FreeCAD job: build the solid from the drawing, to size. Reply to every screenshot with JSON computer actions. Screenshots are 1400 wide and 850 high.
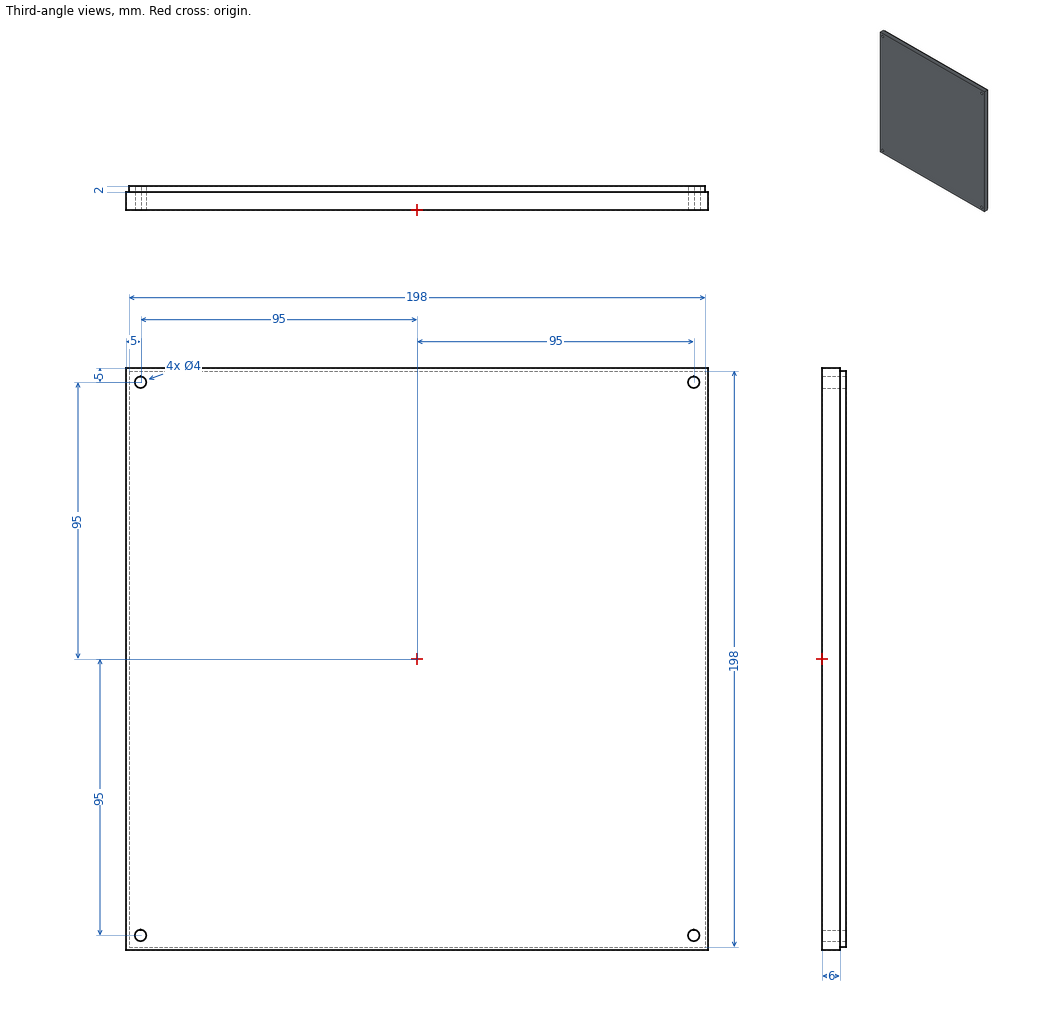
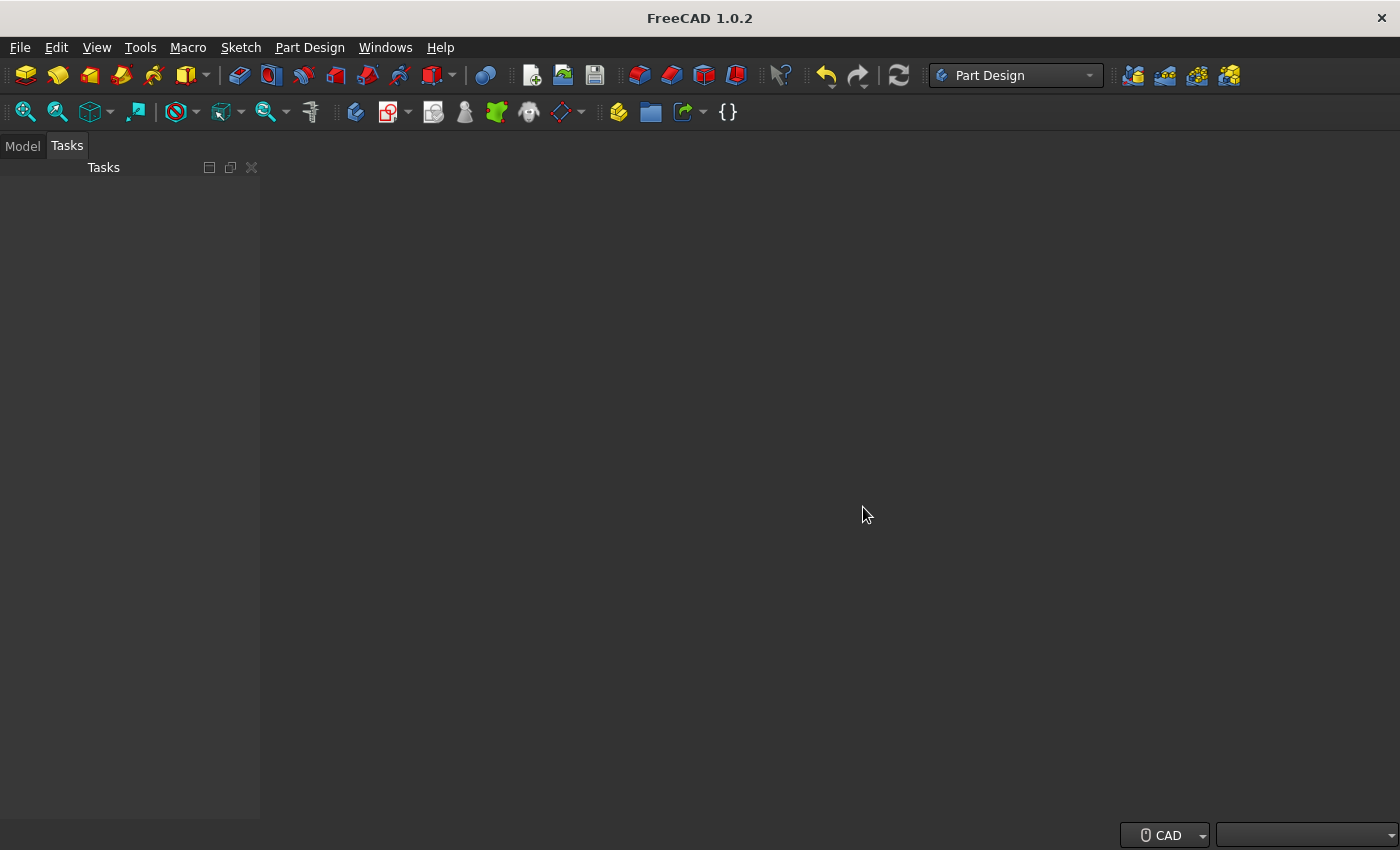
{"action": "left_click", "coordinate": [532, 76]}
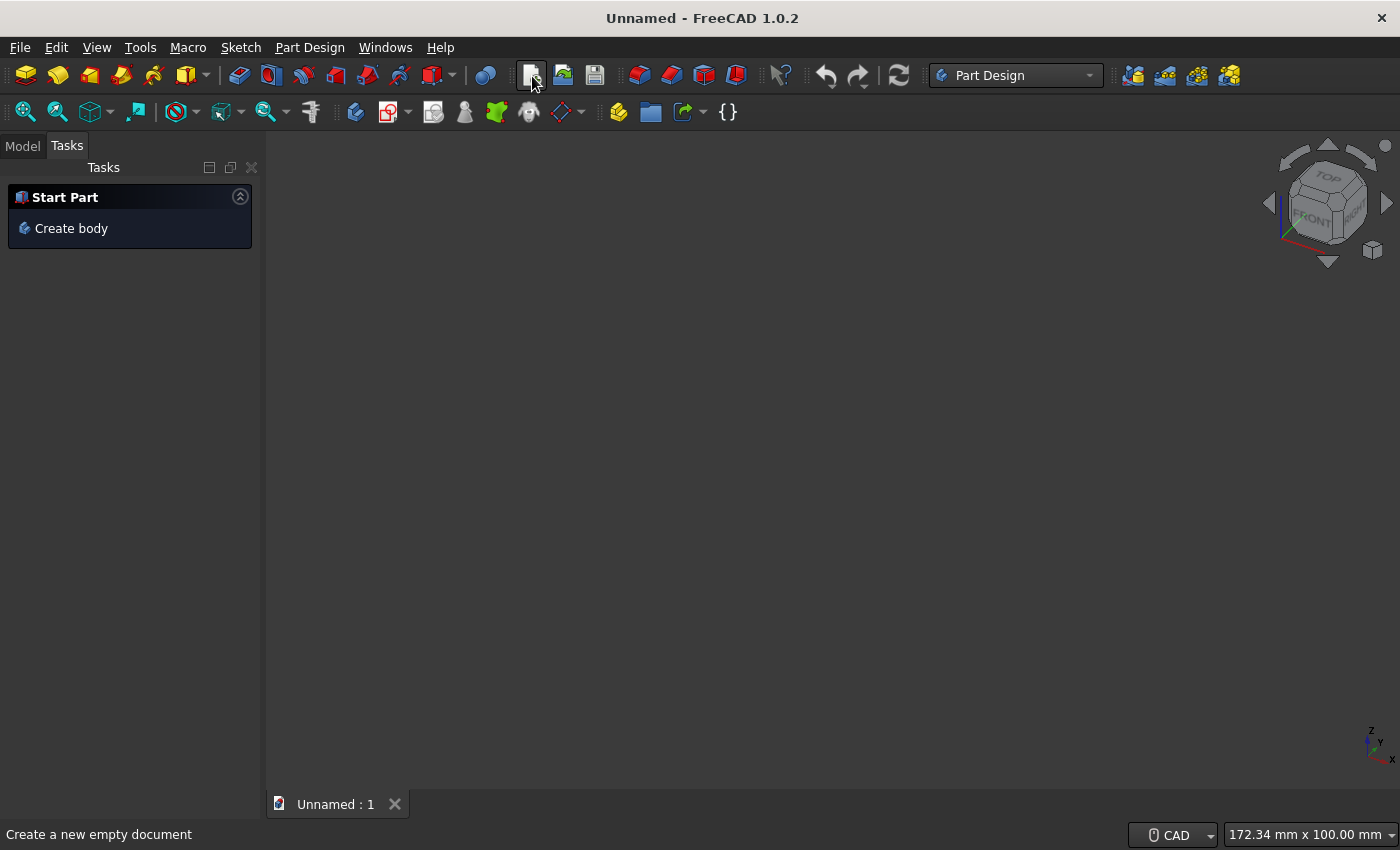
{"action": "left_click", "coordinate": [388, 112]}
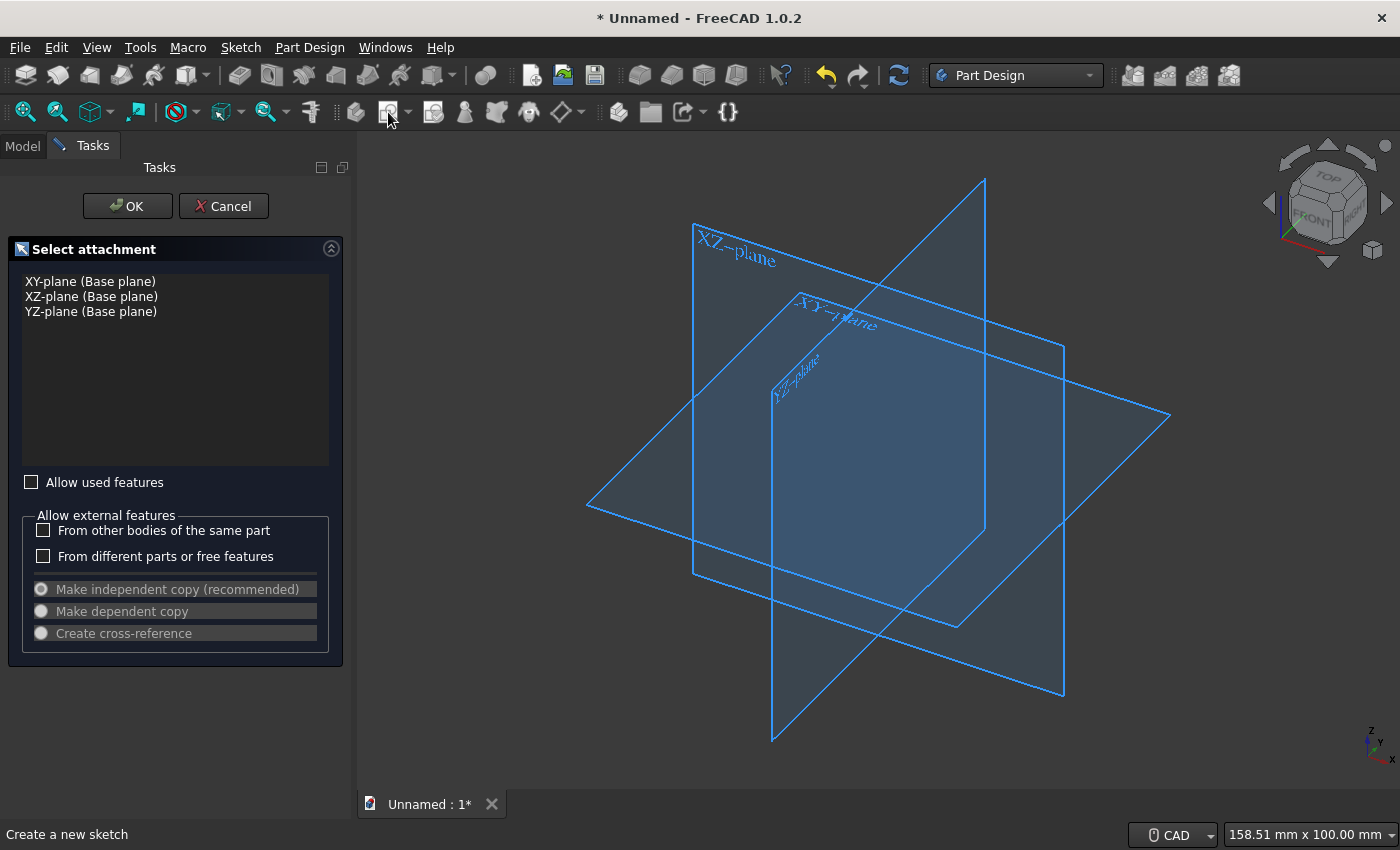
{"action": "left_click", "coordinate": [82, 296]}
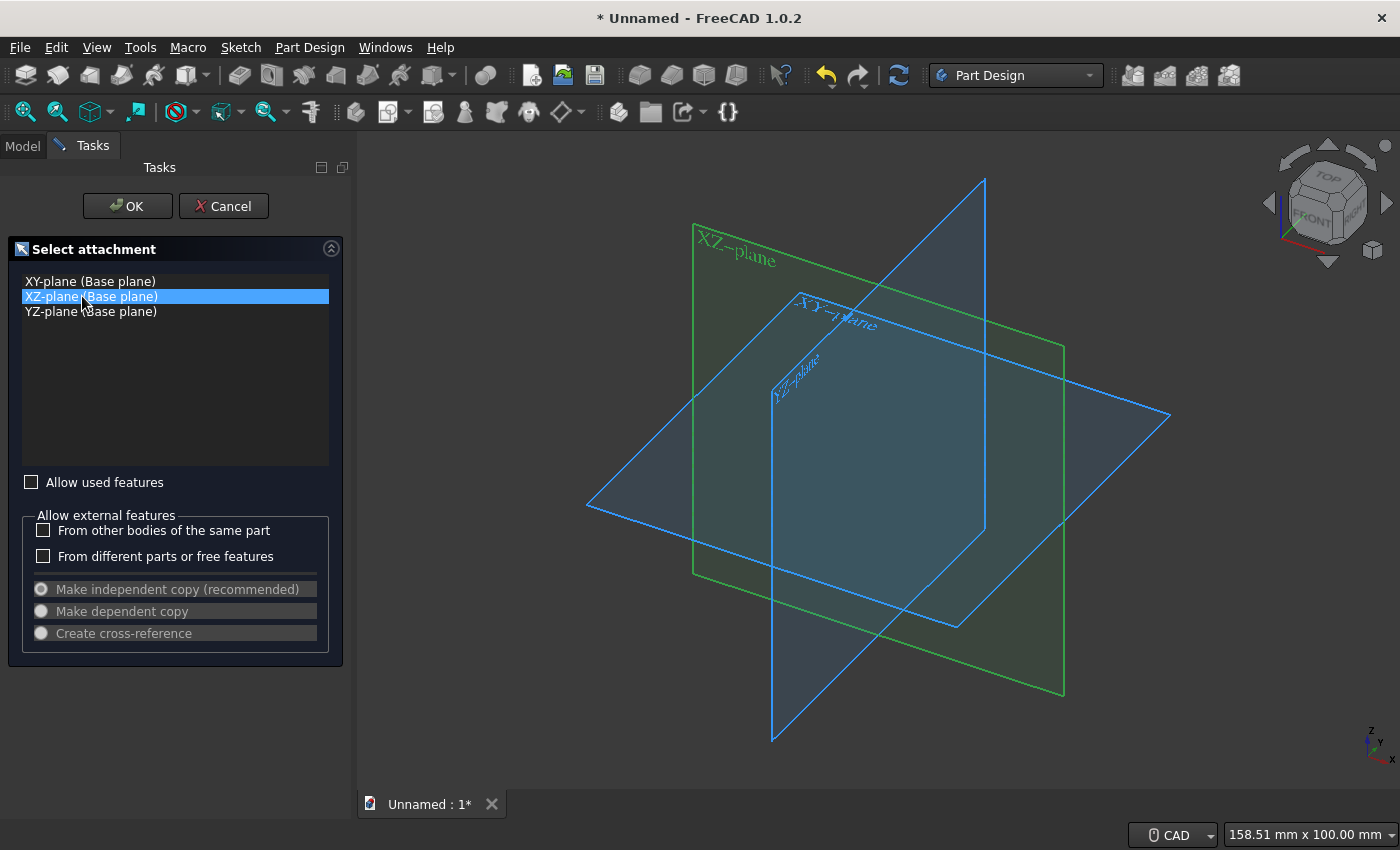
{"action": "left_click", "coordinate": [128, 206]}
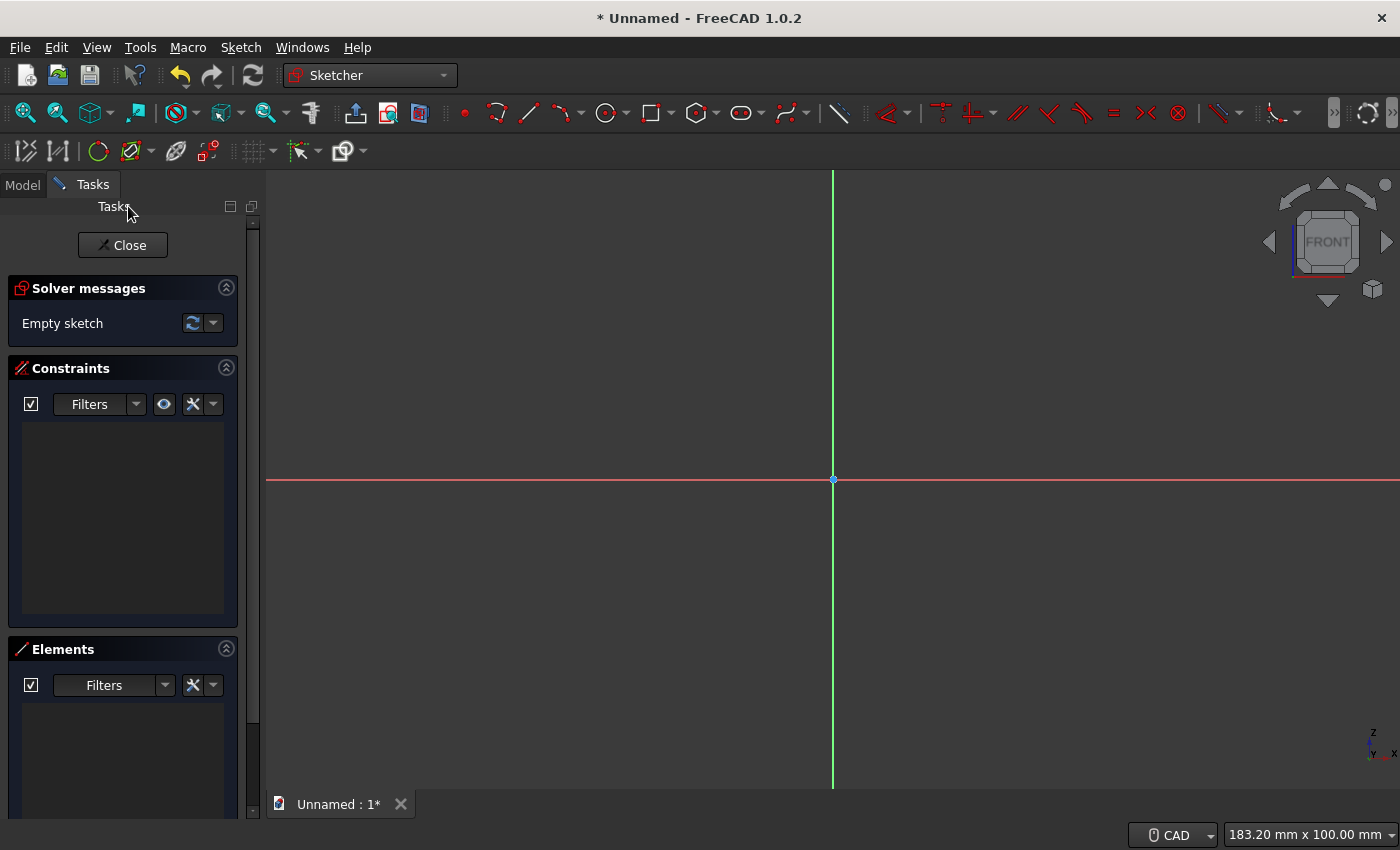
{"action": "scroll", "coordinate": [735, 479], "scroll_direction": "down", "scroll_amount": 6}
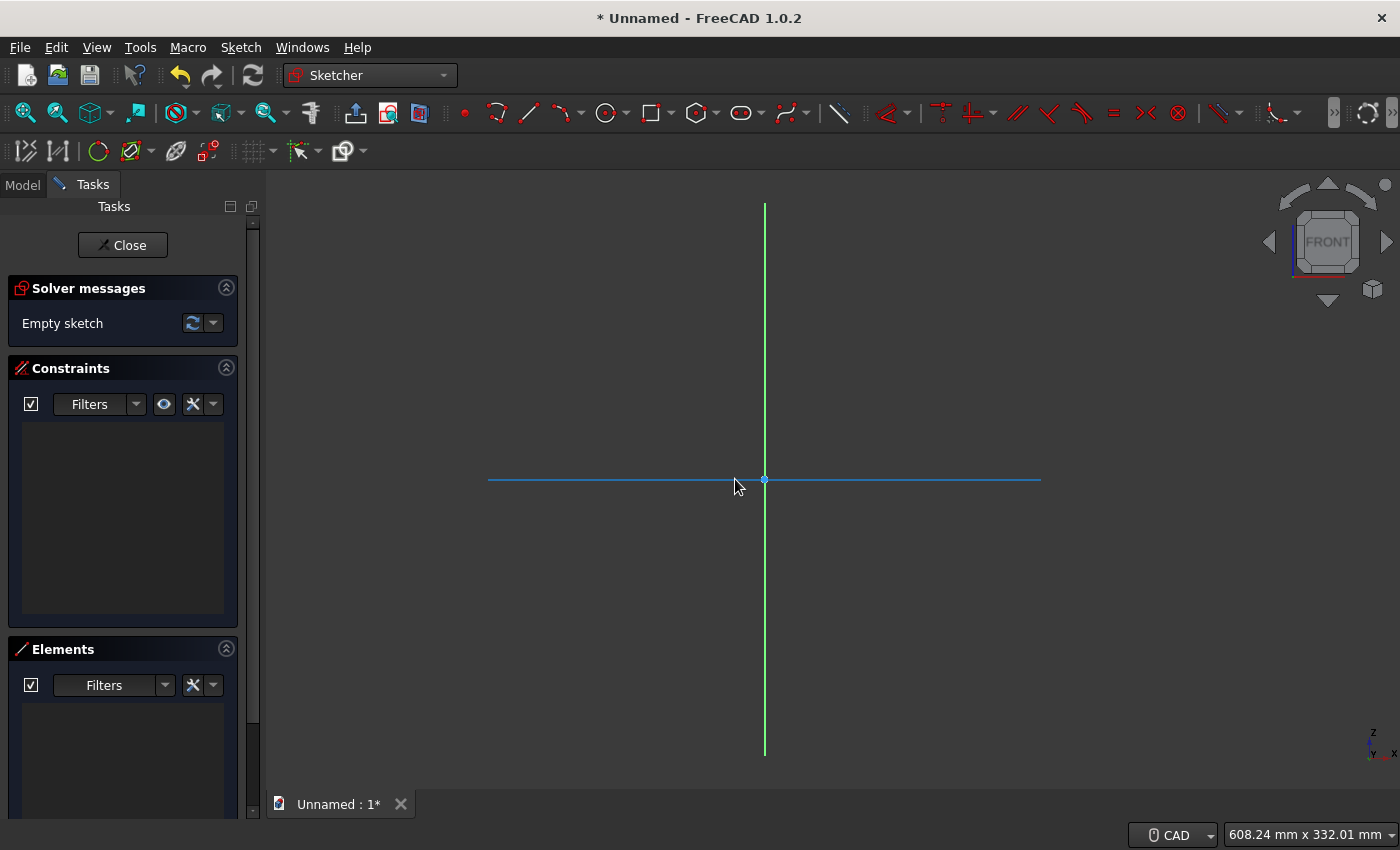
{"action": "left_click", "coordinate": [674, 114]}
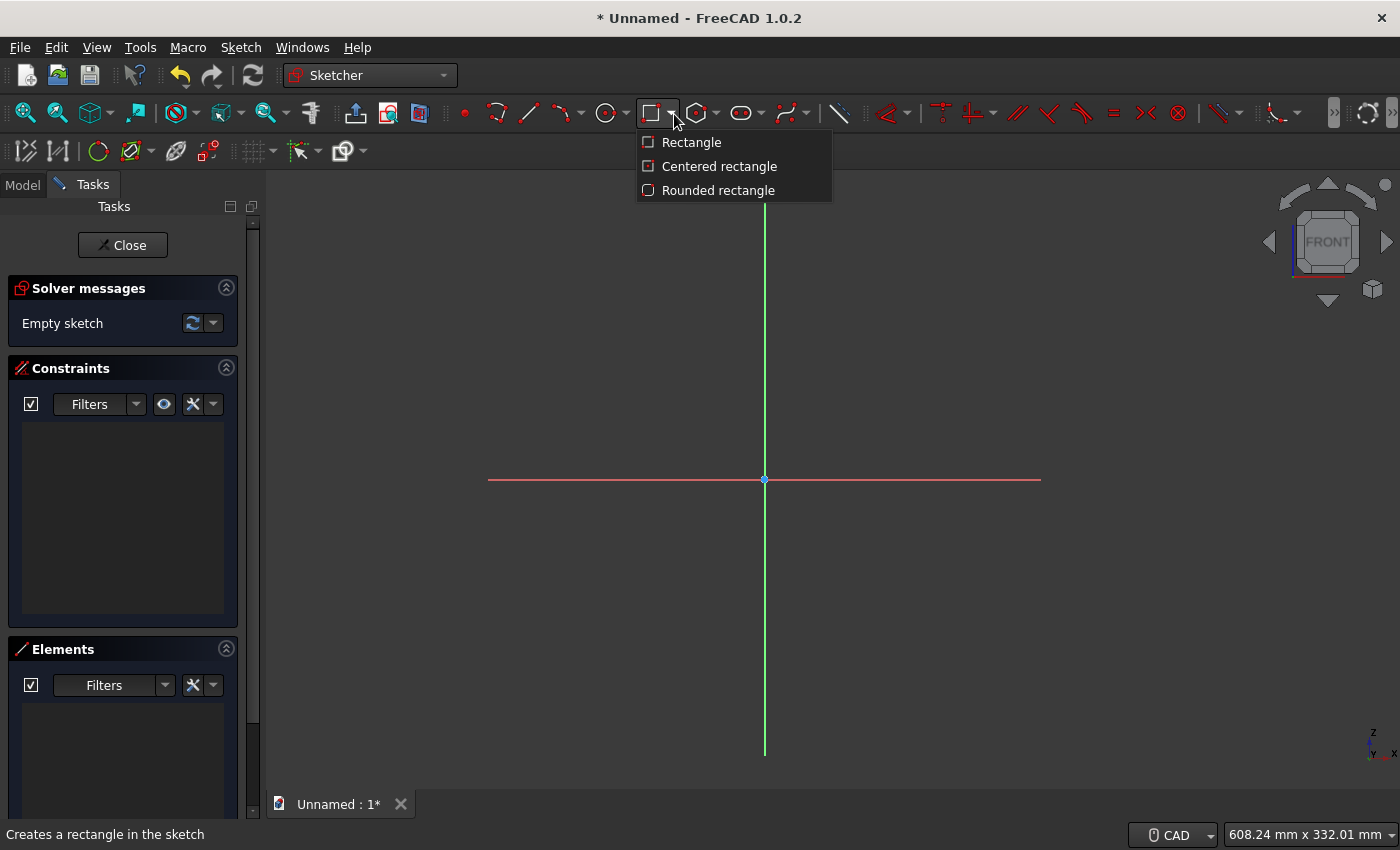
{"action": "left_click", "coordinate": [734, 166]}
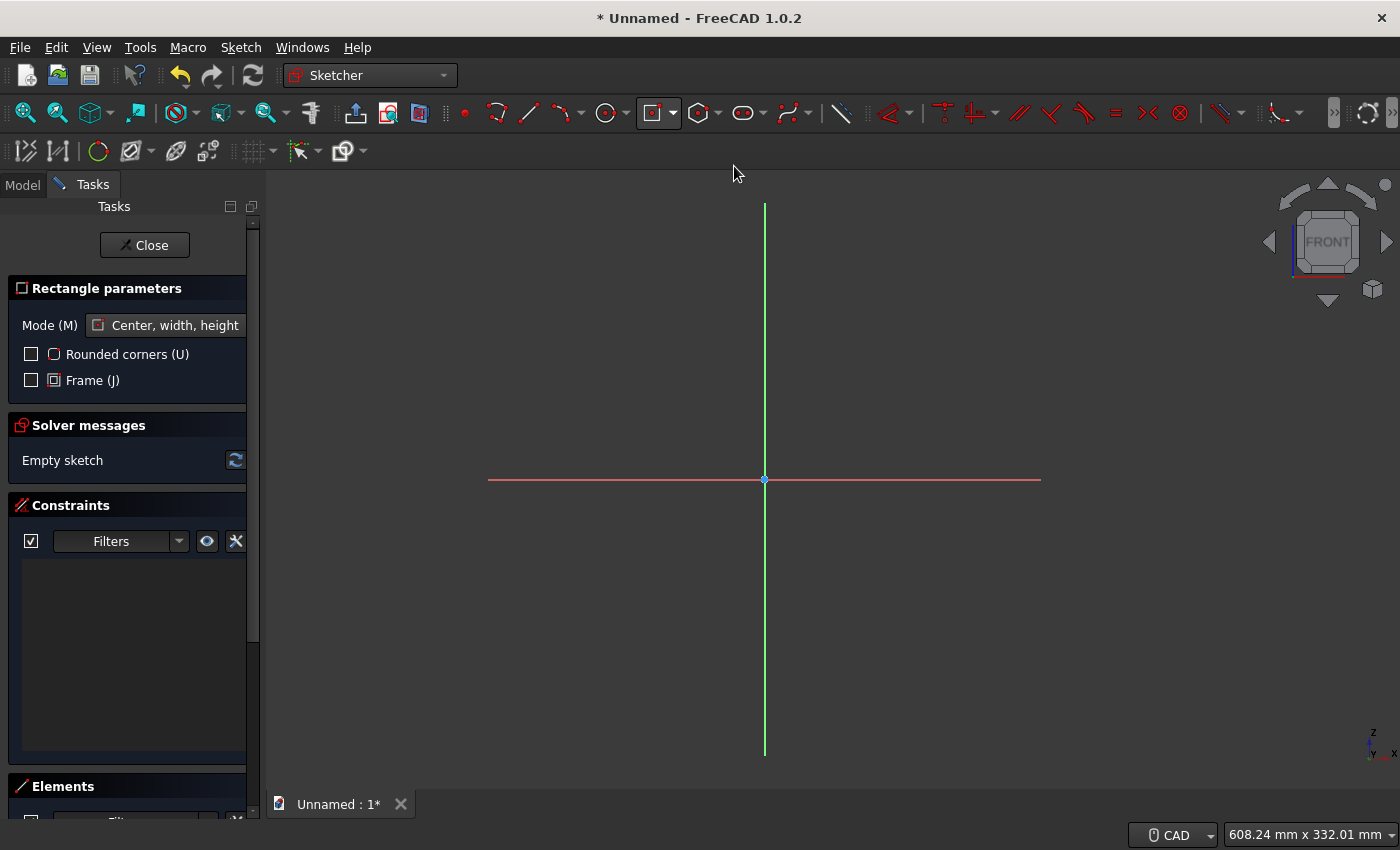
{"action": "left_click", "coordinate": [765, 480]}
{"action": "left_click", "coordinate": [951, 293]}